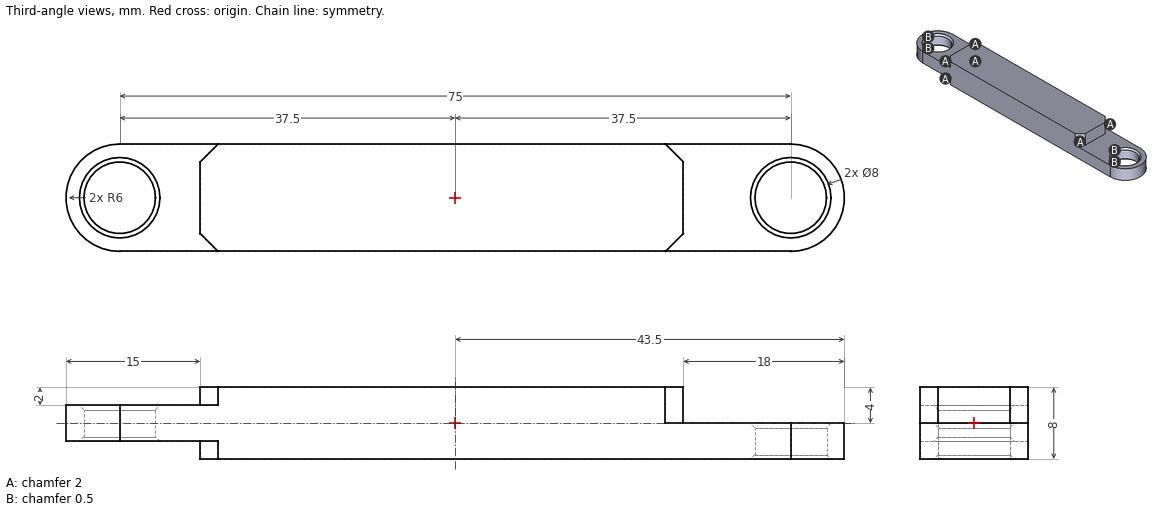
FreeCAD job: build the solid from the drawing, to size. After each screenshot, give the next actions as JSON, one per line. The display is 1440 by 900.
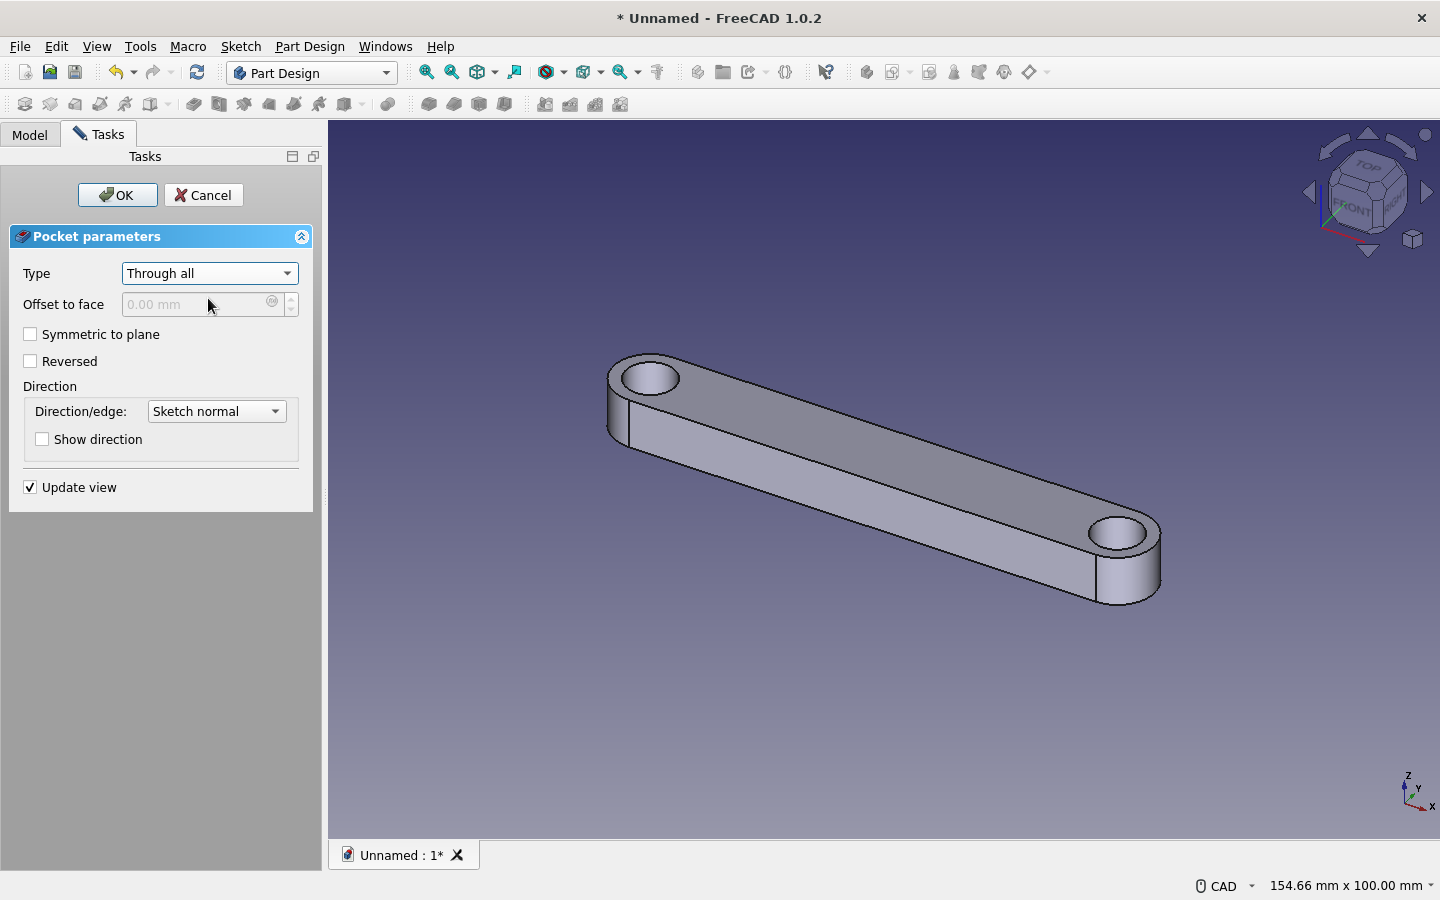
{"action": "left_click", "coordinate": [118, 195]}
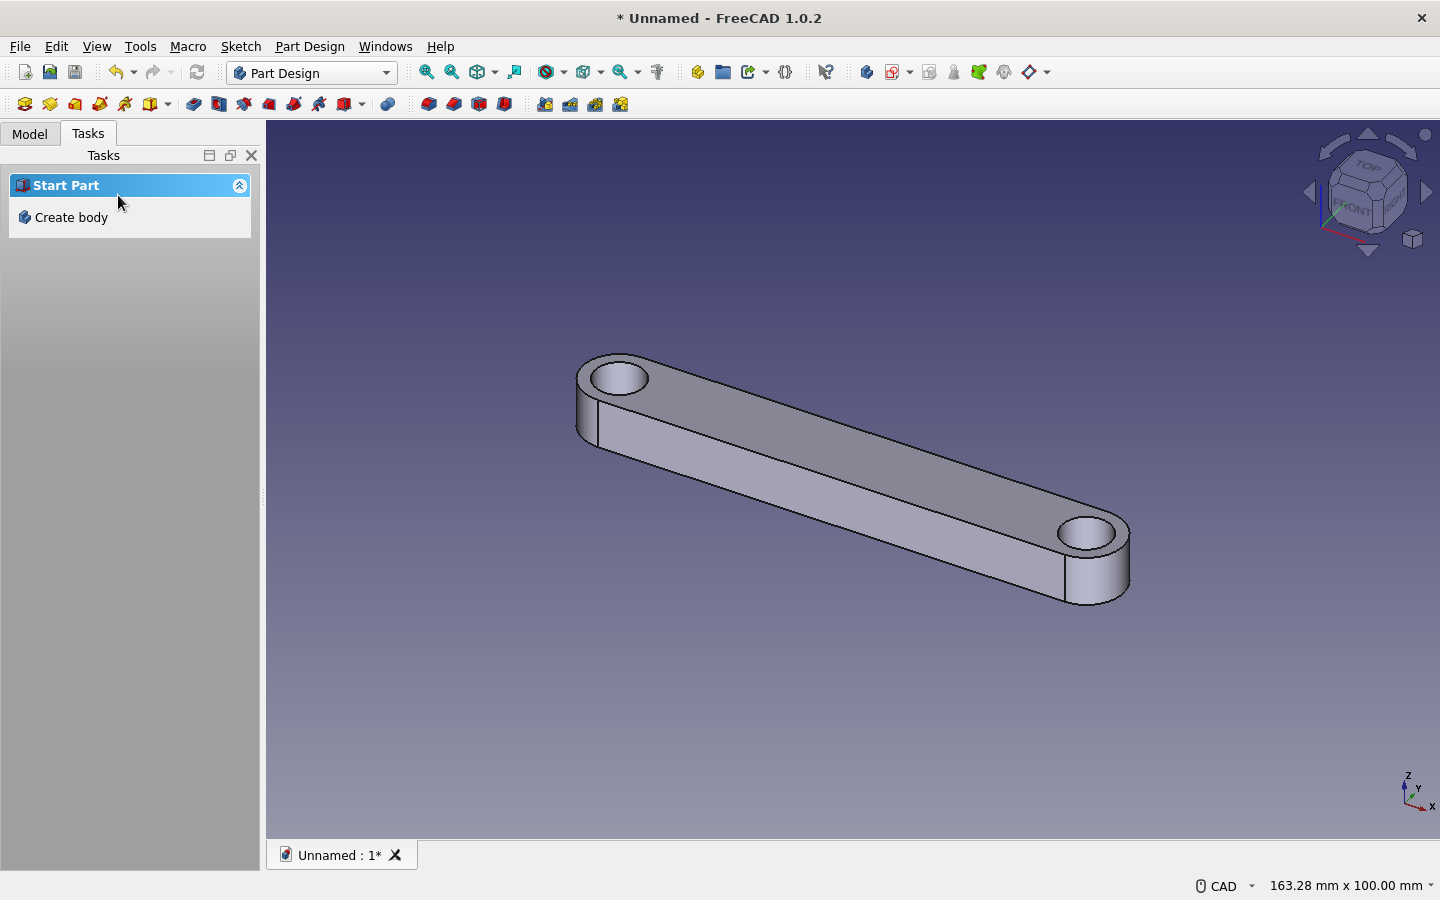
{"action": "key", "text": "4"}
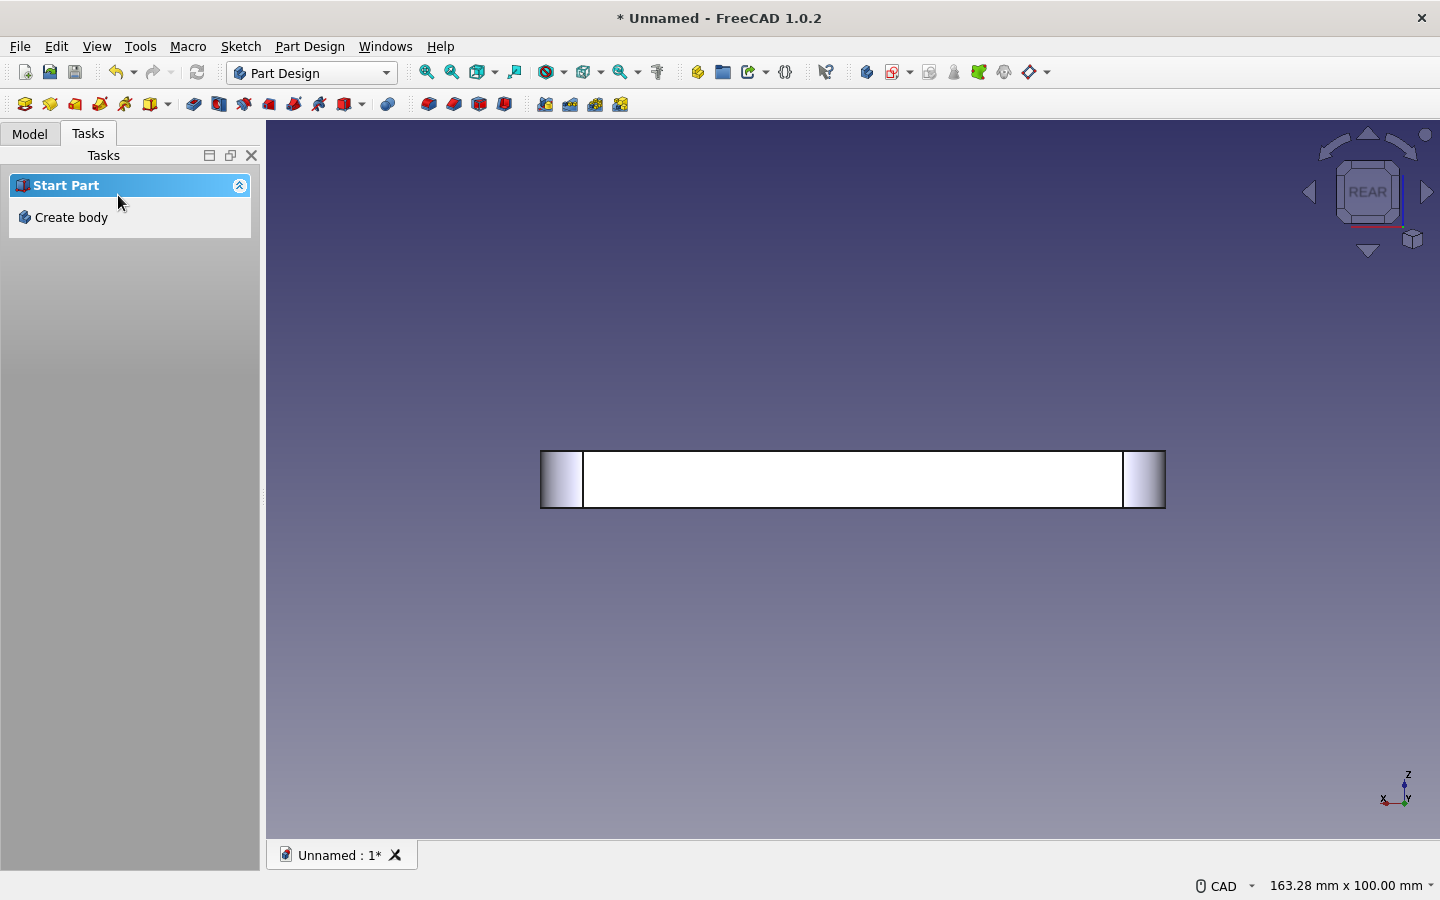
{"action": "left_click", "coordinate": [622, 478]}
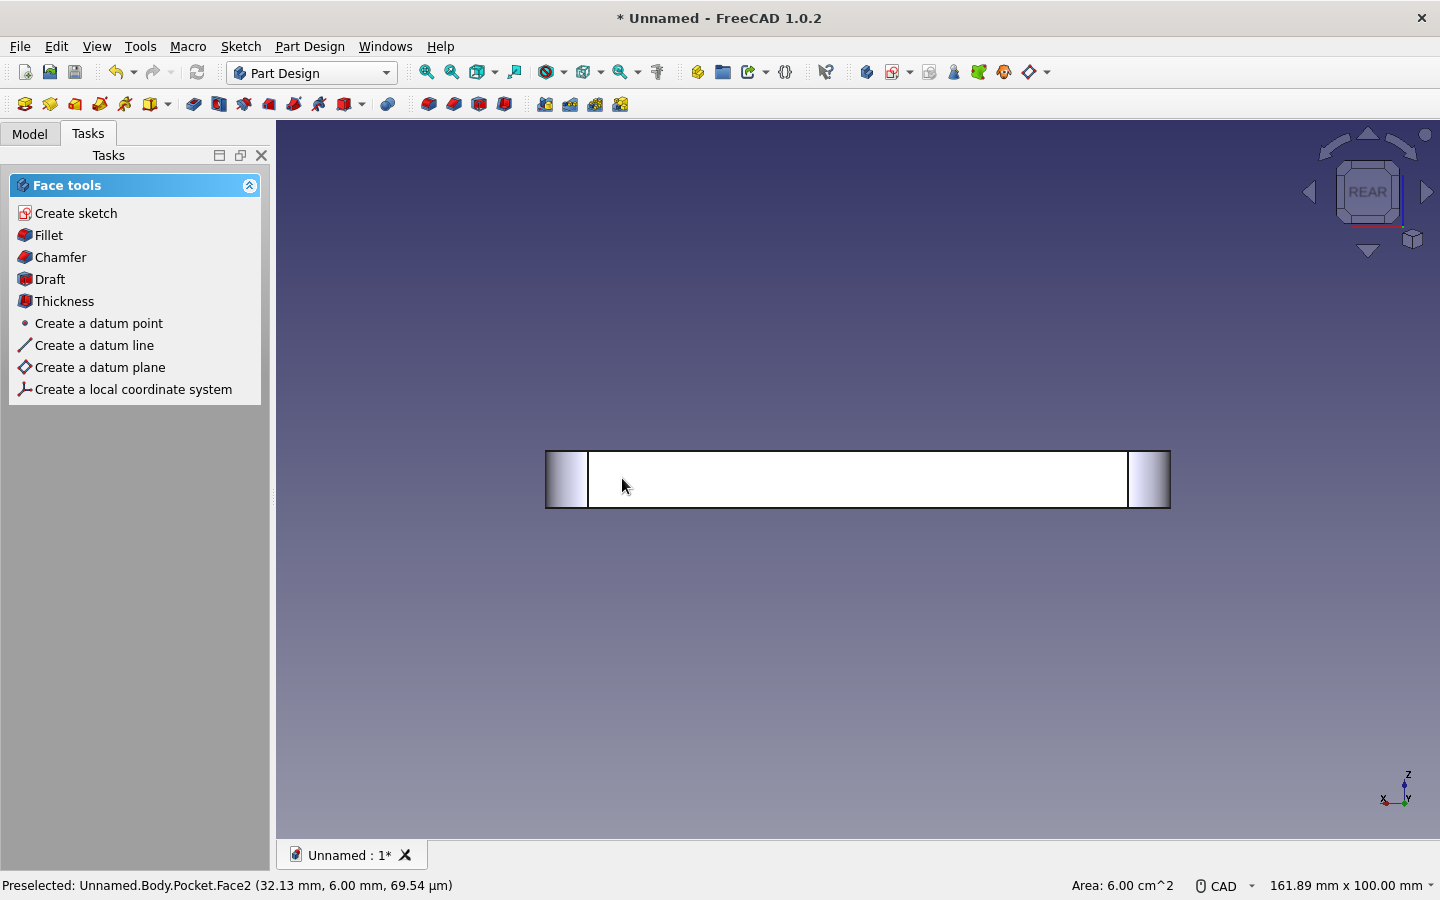
{"action": "left_click", "coordinate": [892, 72]}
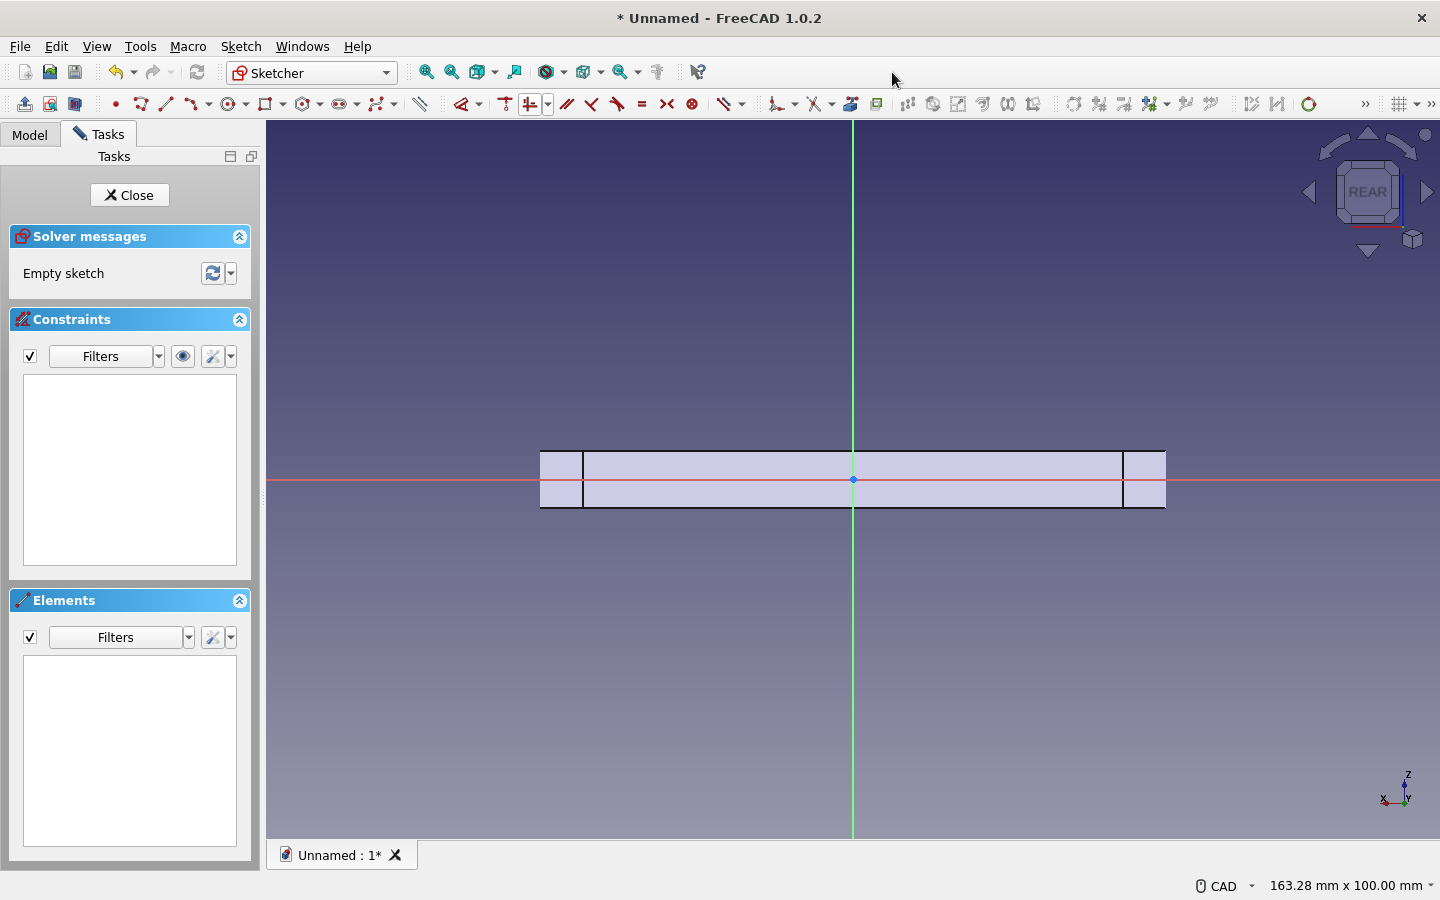
{"action": "left_click", "coordinate": [264, 104]}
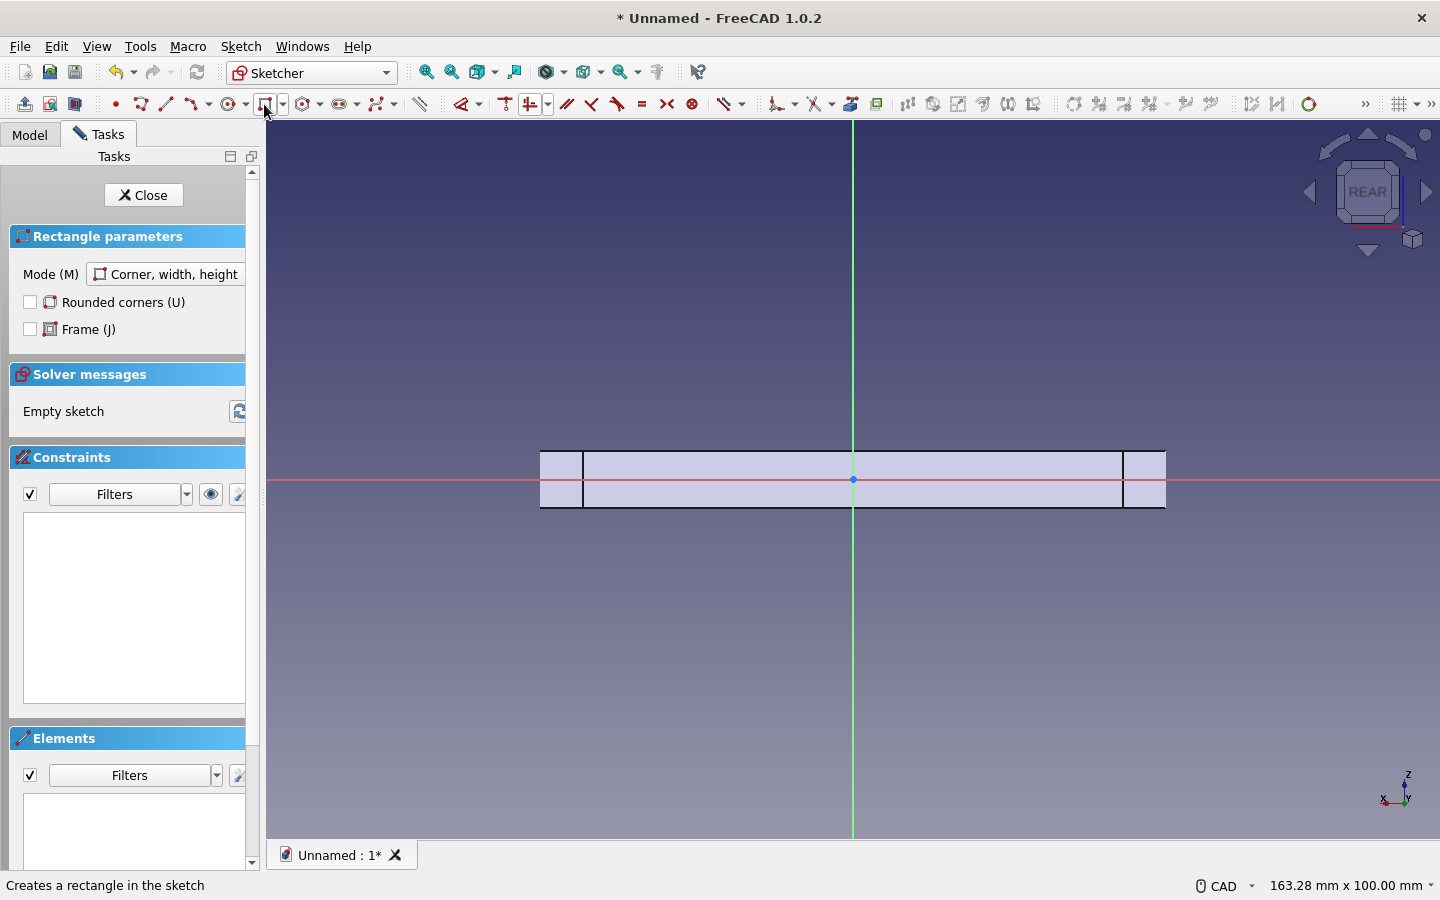
{"action": "left_click", "coordinate": [540, 451]}
{"action": "left_click", "coordinate": [670, 479]}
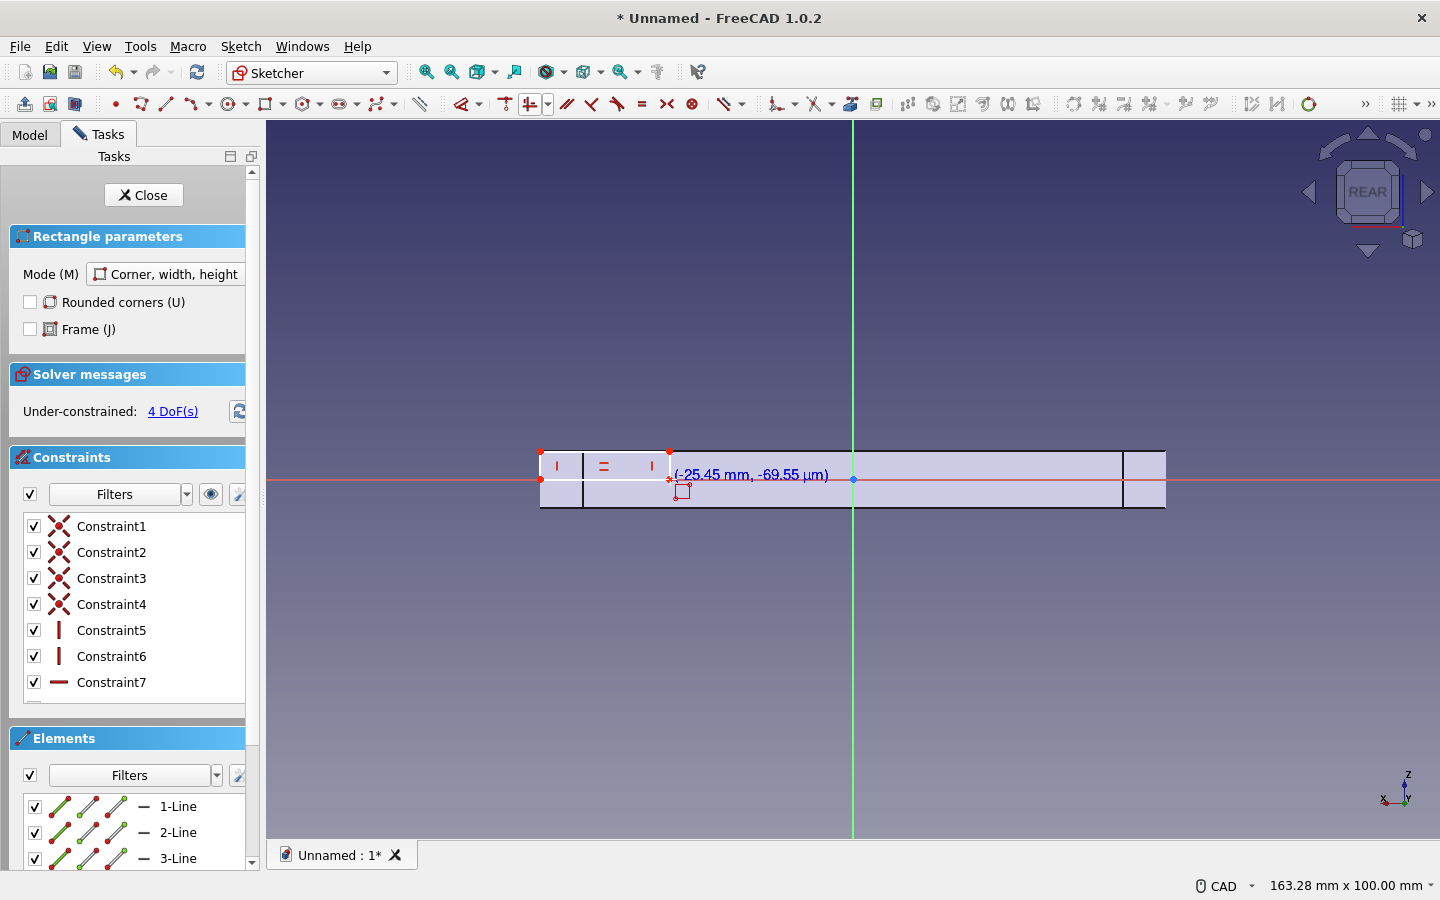
{"action": "left_click", "coordinate": [1058, 451]}
{"action": "left_click", "coordinate": [1166, 465]}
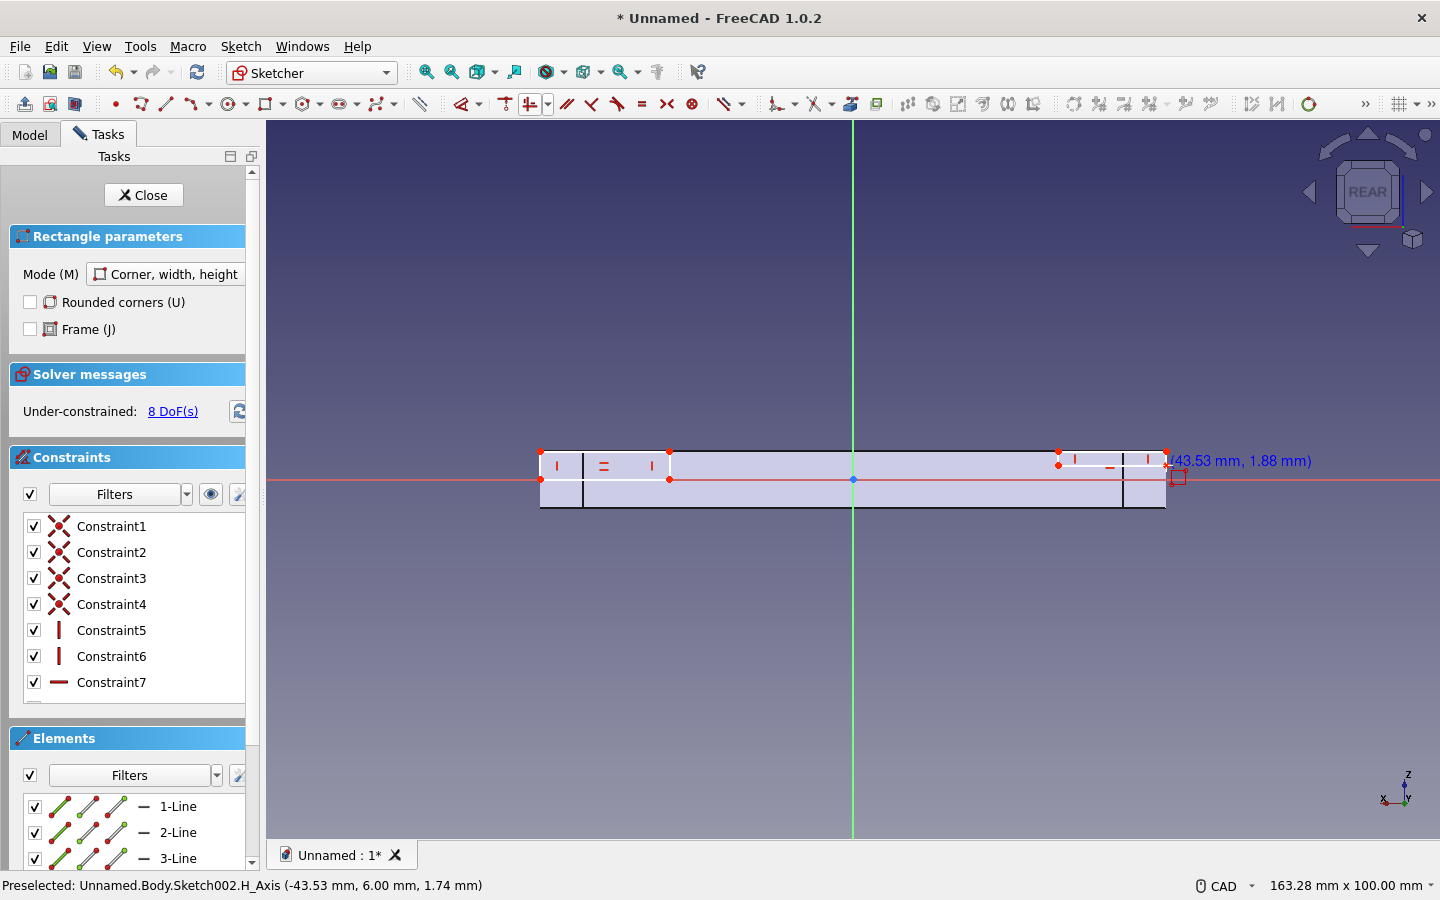
{"action": "left_click", "coordinate": [1058, 494]}
{"action": "left_click", "coordinate": [1166, 508]}
{"action": "key", "text": "Escape"}